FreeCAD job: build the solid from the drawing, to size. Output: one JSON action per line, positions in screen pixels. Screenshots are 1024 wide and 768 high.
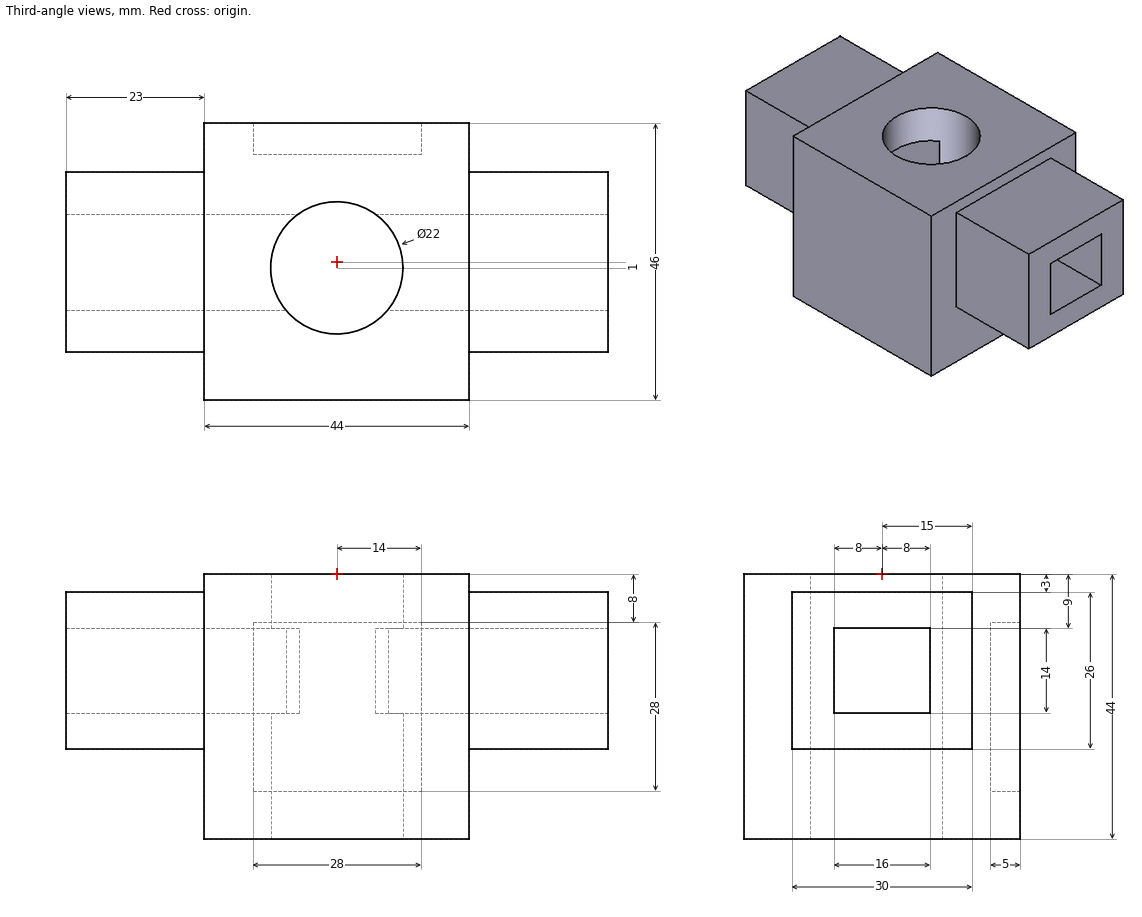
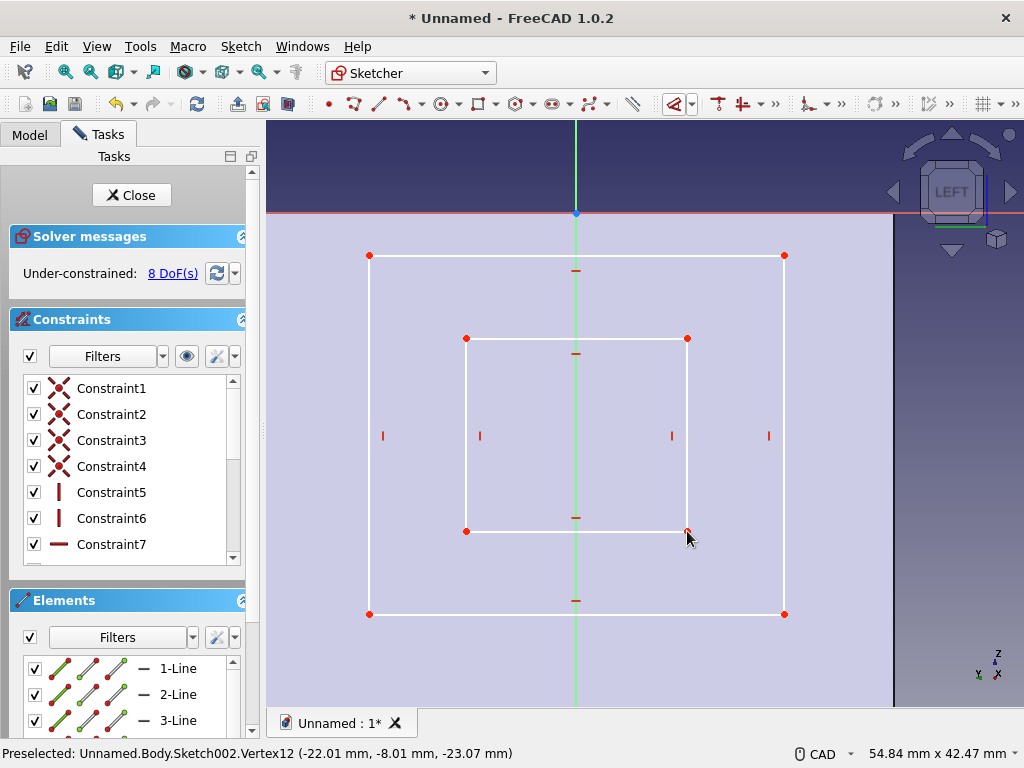
{"action": "left_click", "coordinate": [369, 364]}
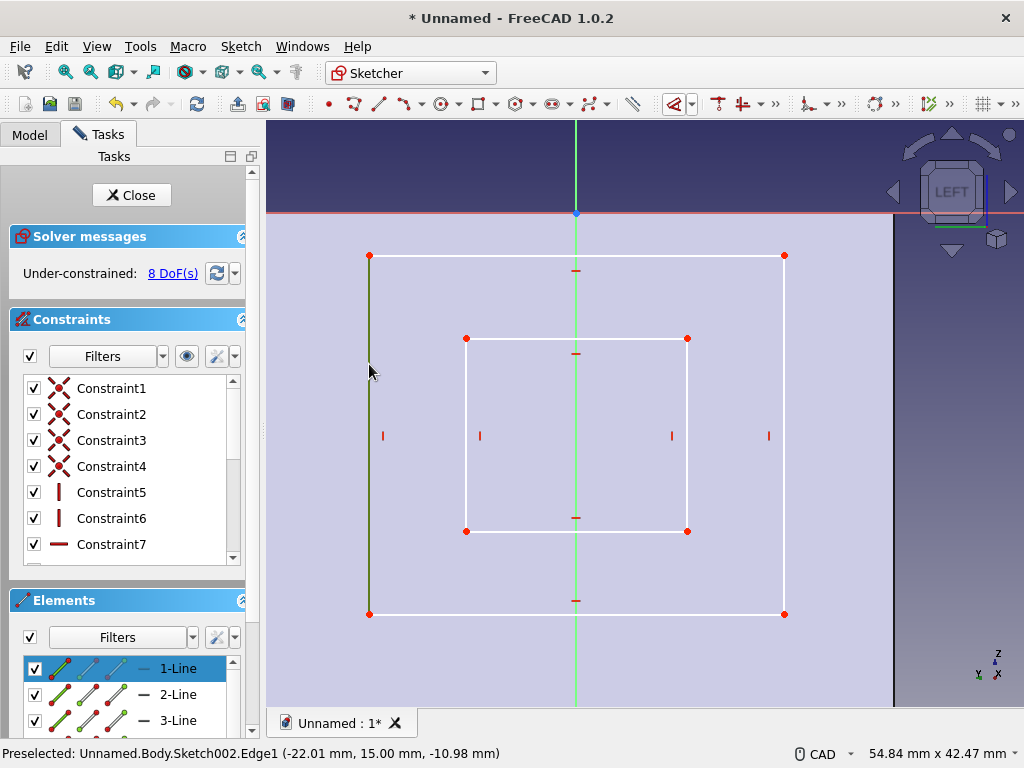
{"action": "key", "text": "i"}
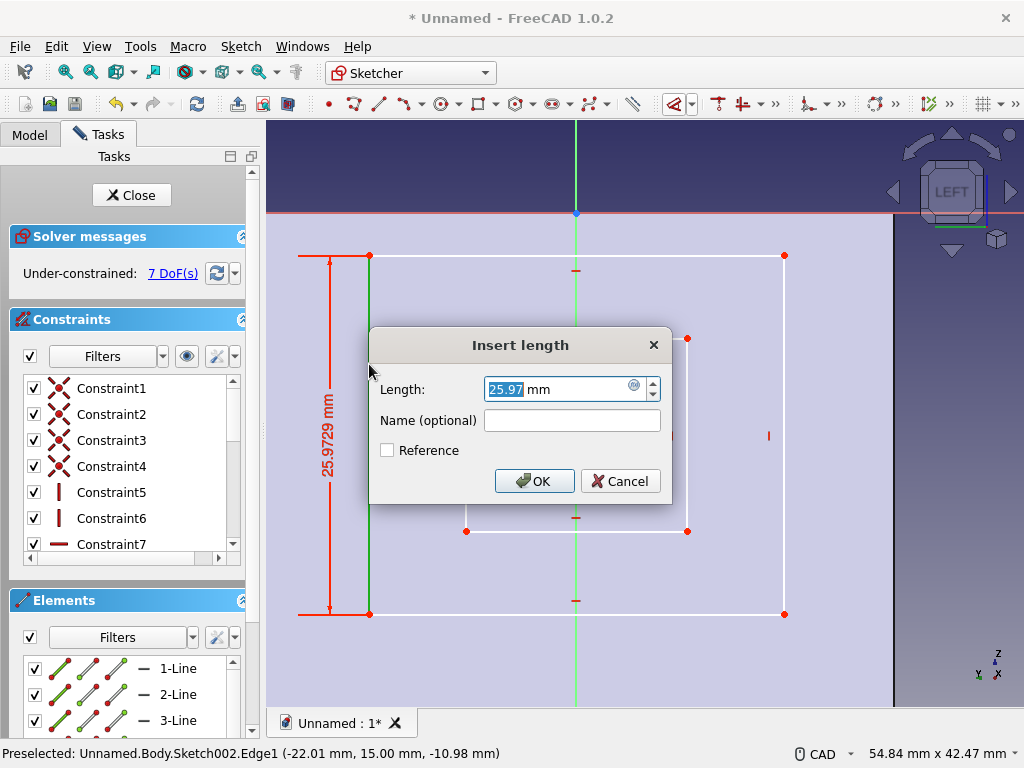
{"action": "type", "text": "26"}
{"action": "key", "text": "Return"}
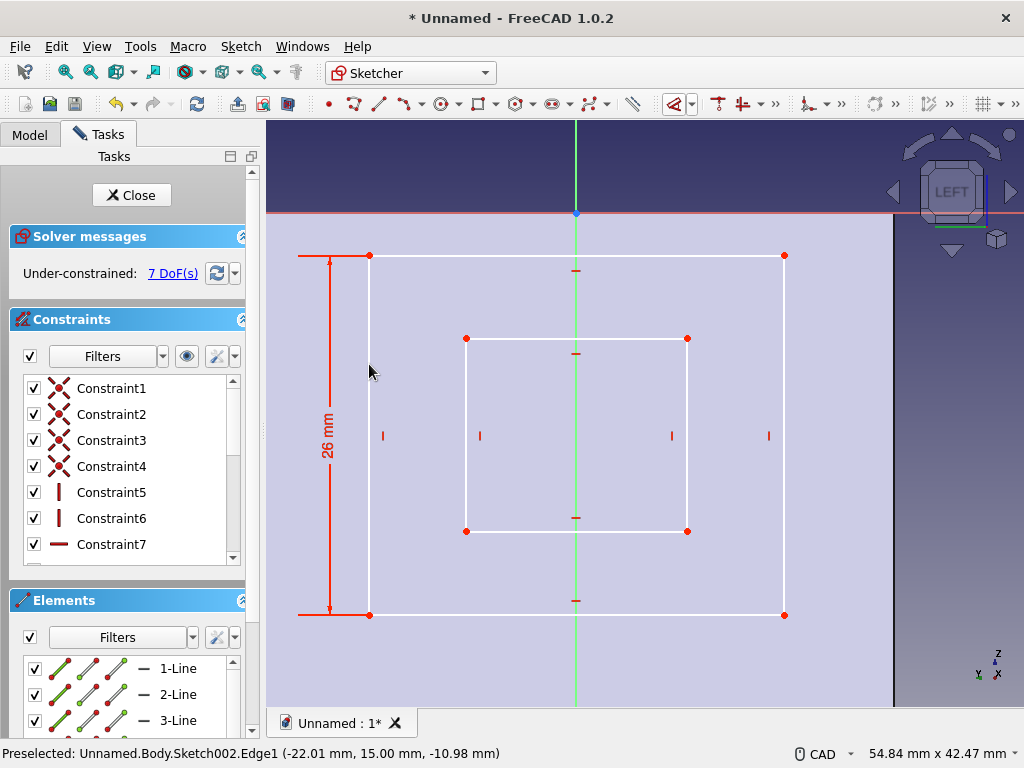
{"action": "left_click", "coordinate": [494, 615]}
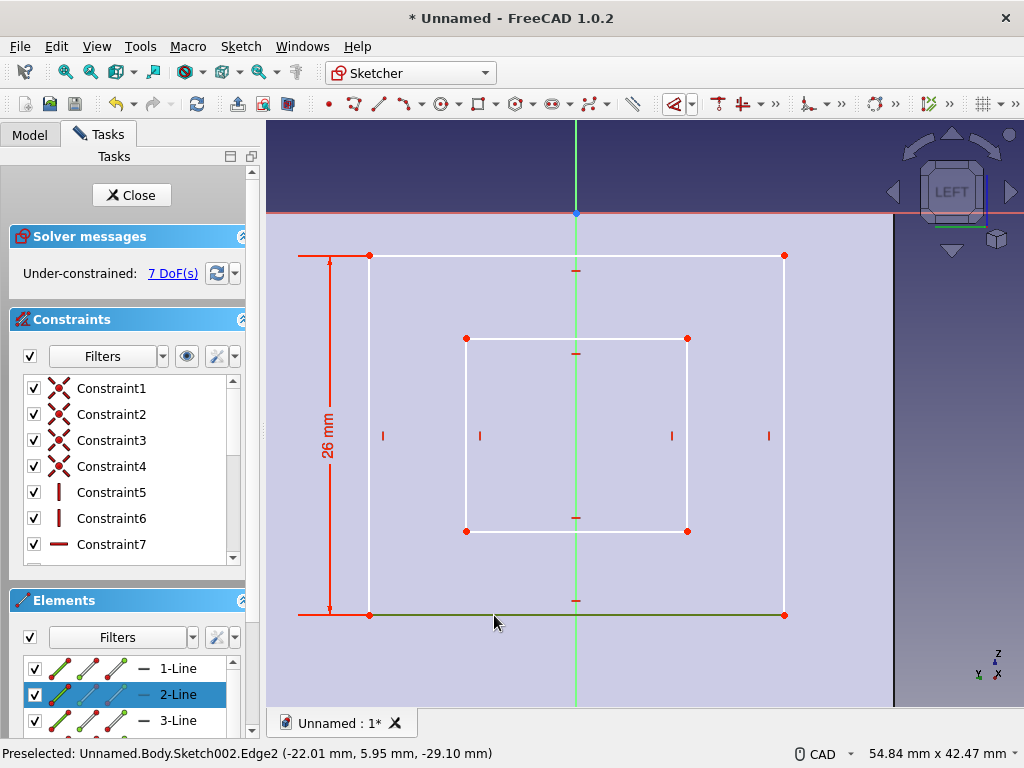
{"action": "key", "text": "l"}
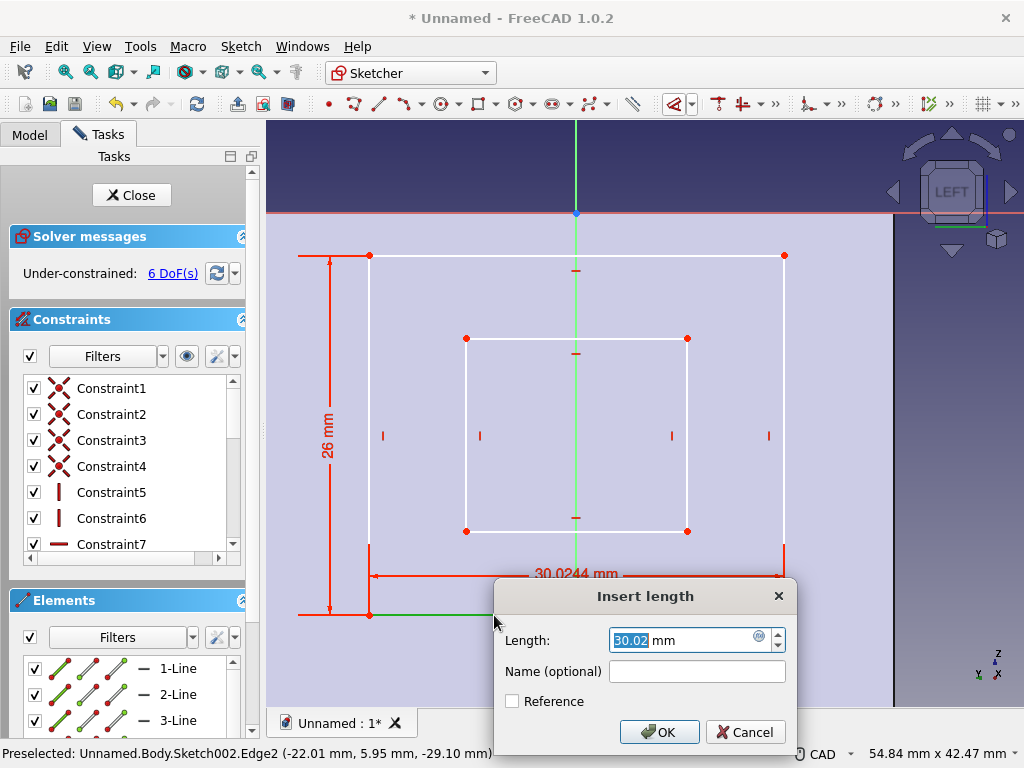
{"action": "type", "text": "30"}
{"action": "key", "text": "Return"}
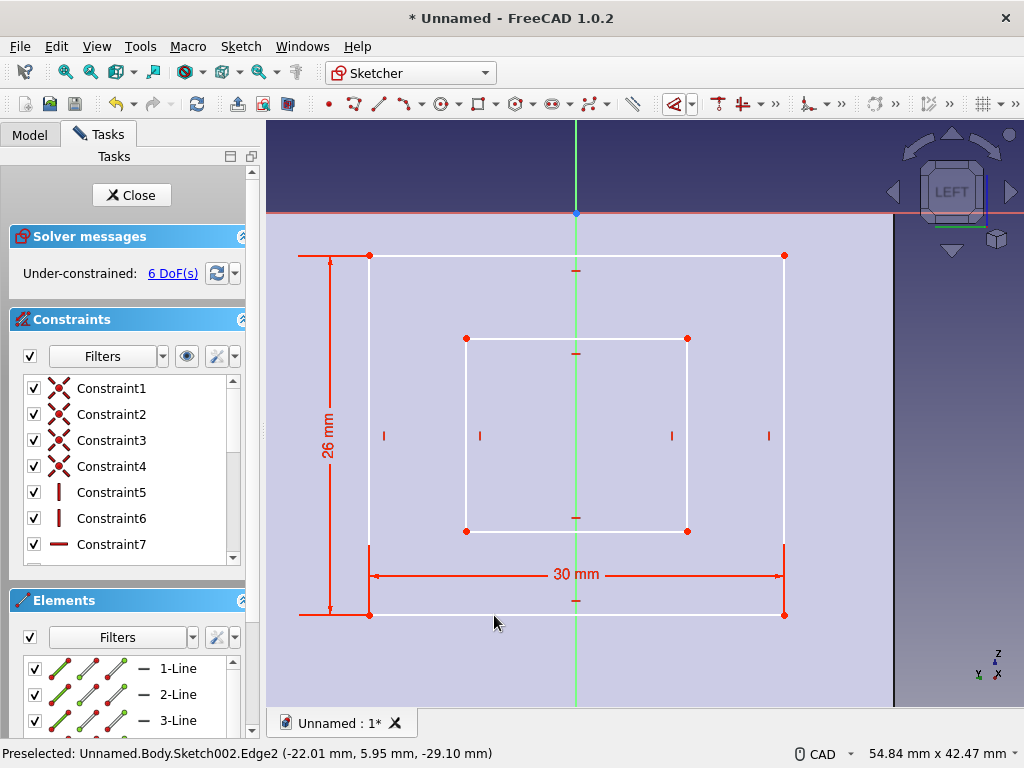
{"action": "left_click", "coordinate": [466, 397]}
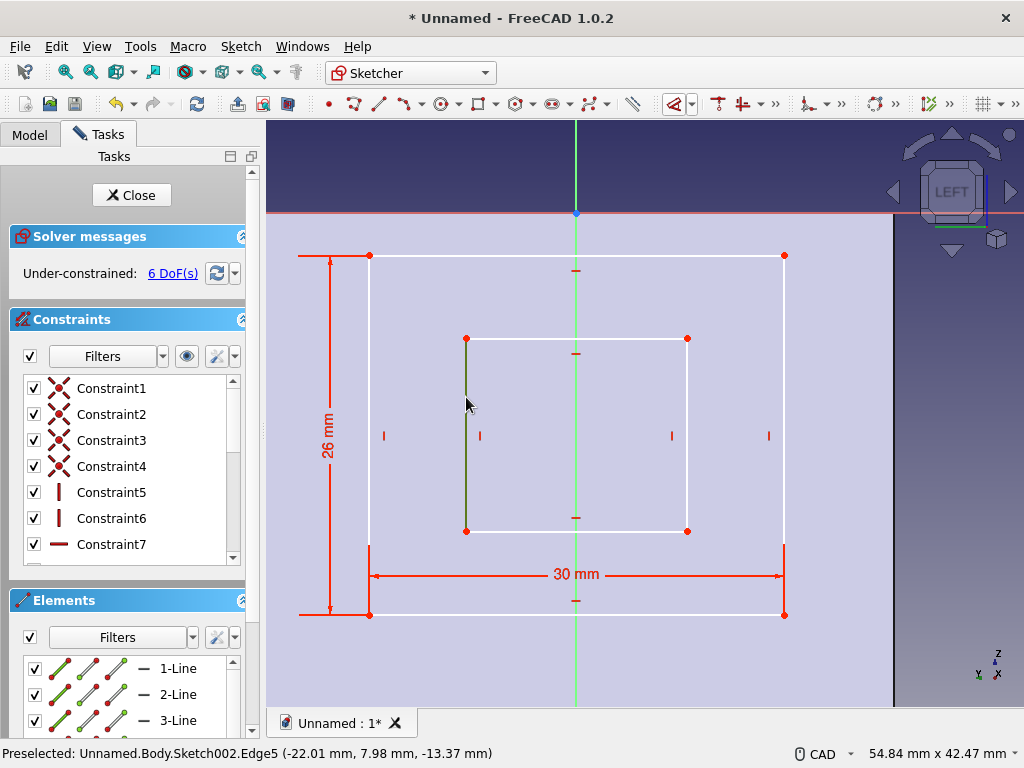
{"action": "key", "text": "i"}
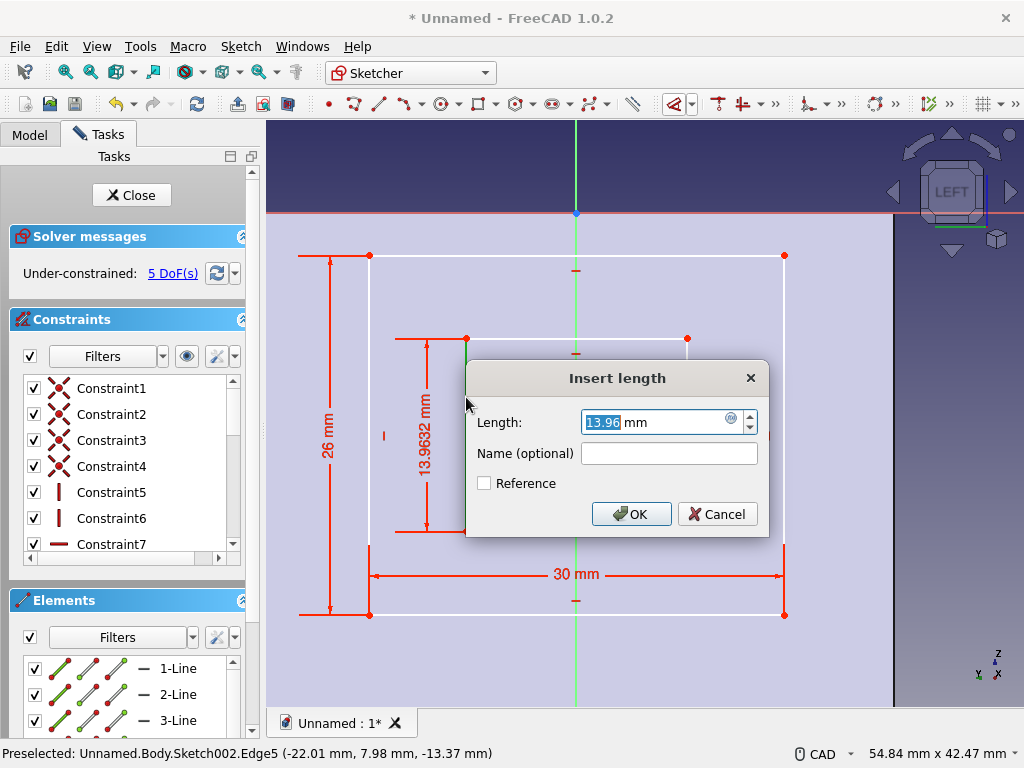
{"action": "type", "text": "14"}
{"action": "key", "text": "Return"}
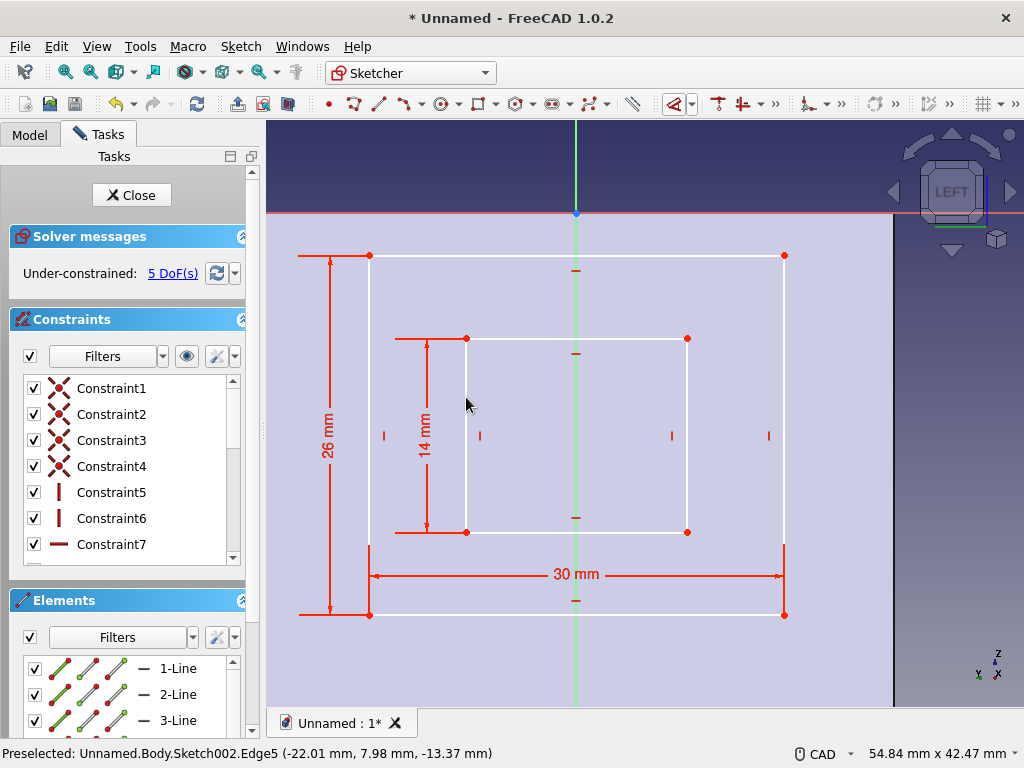
{"action": "left_click", "coordinate": [532, 533]}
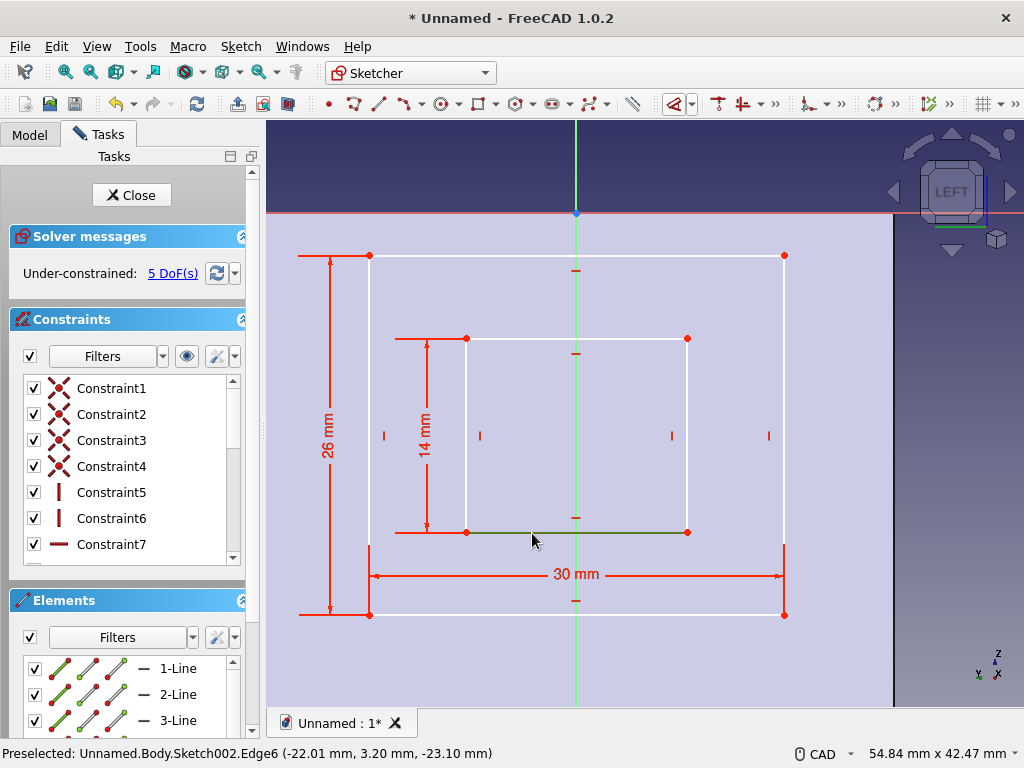
{"action": "key", "text": "l"}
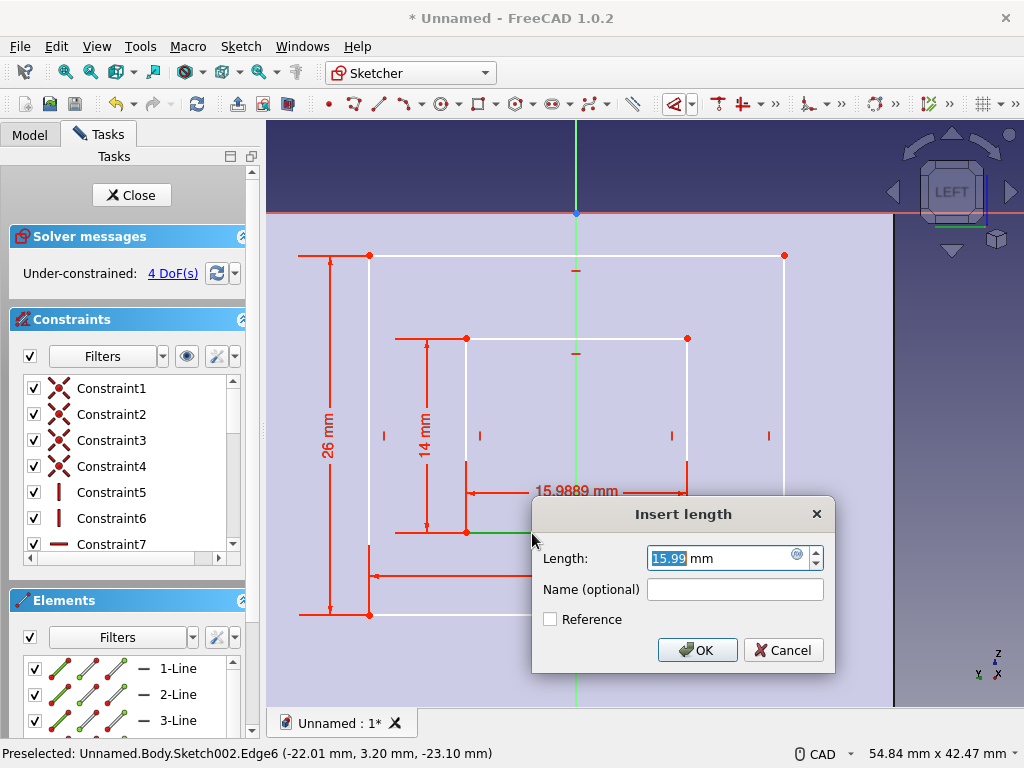
{"action": "type", "text": "16"}
{"action": "key", "text": "Return"}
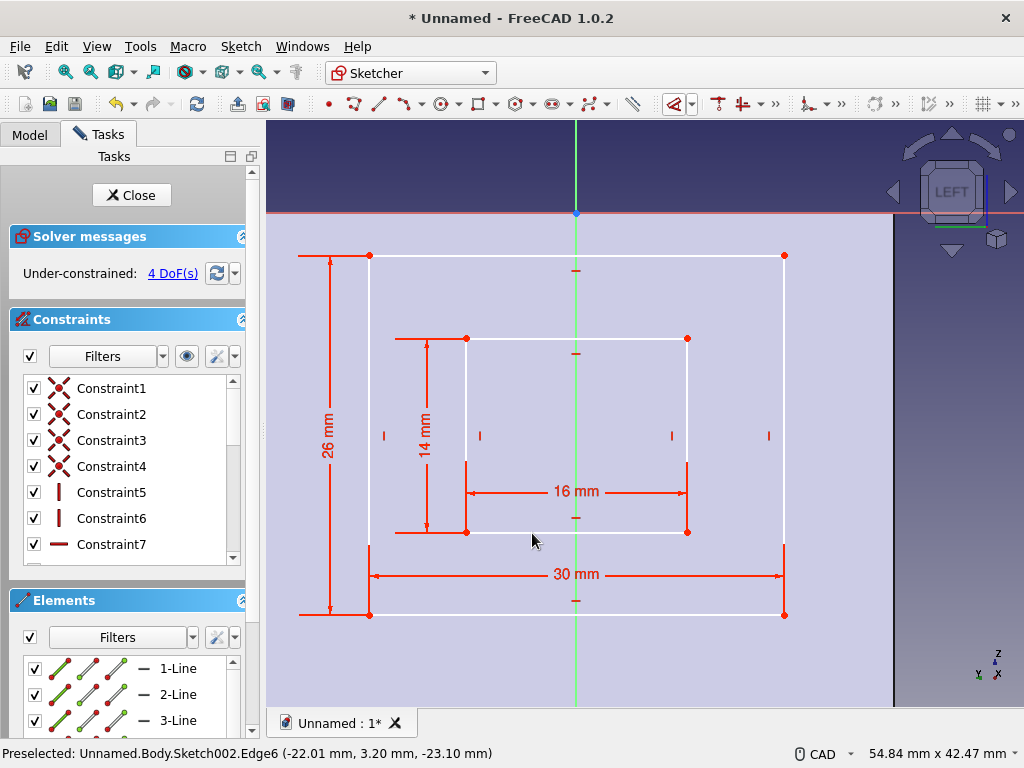
{"action": "left_click", "coordinate": [369, 256]}